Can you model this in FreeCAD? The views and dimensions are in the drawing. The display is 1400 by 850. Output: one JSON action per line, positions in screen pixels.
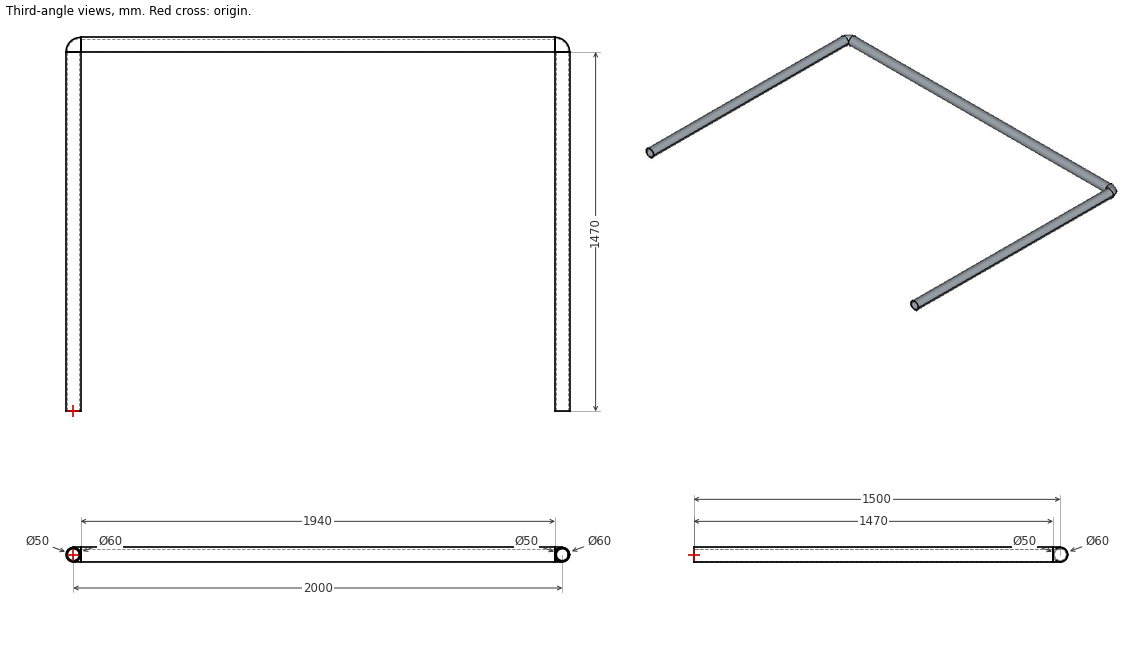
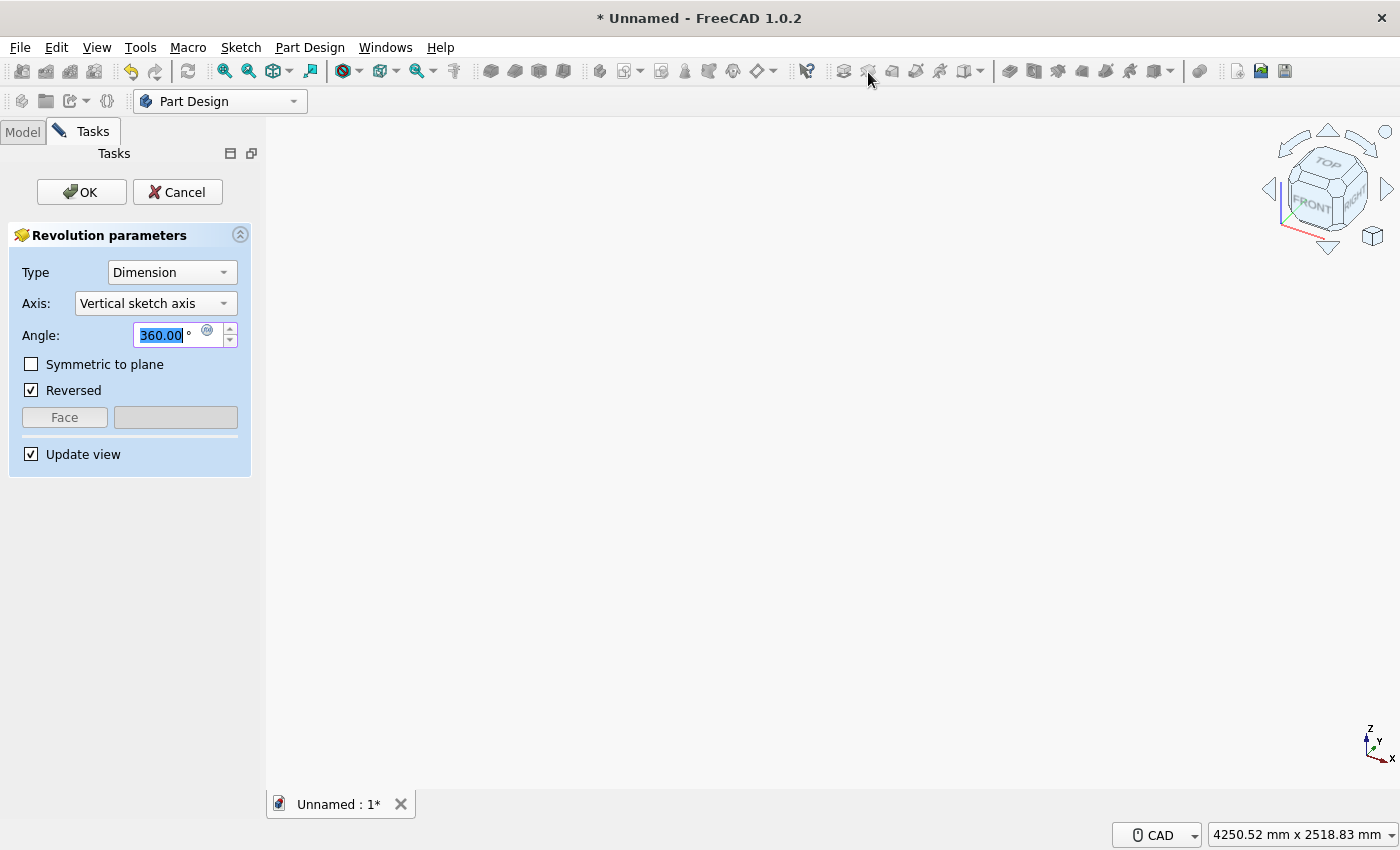
{"action": "left_click", "coordinate": [156, 304]}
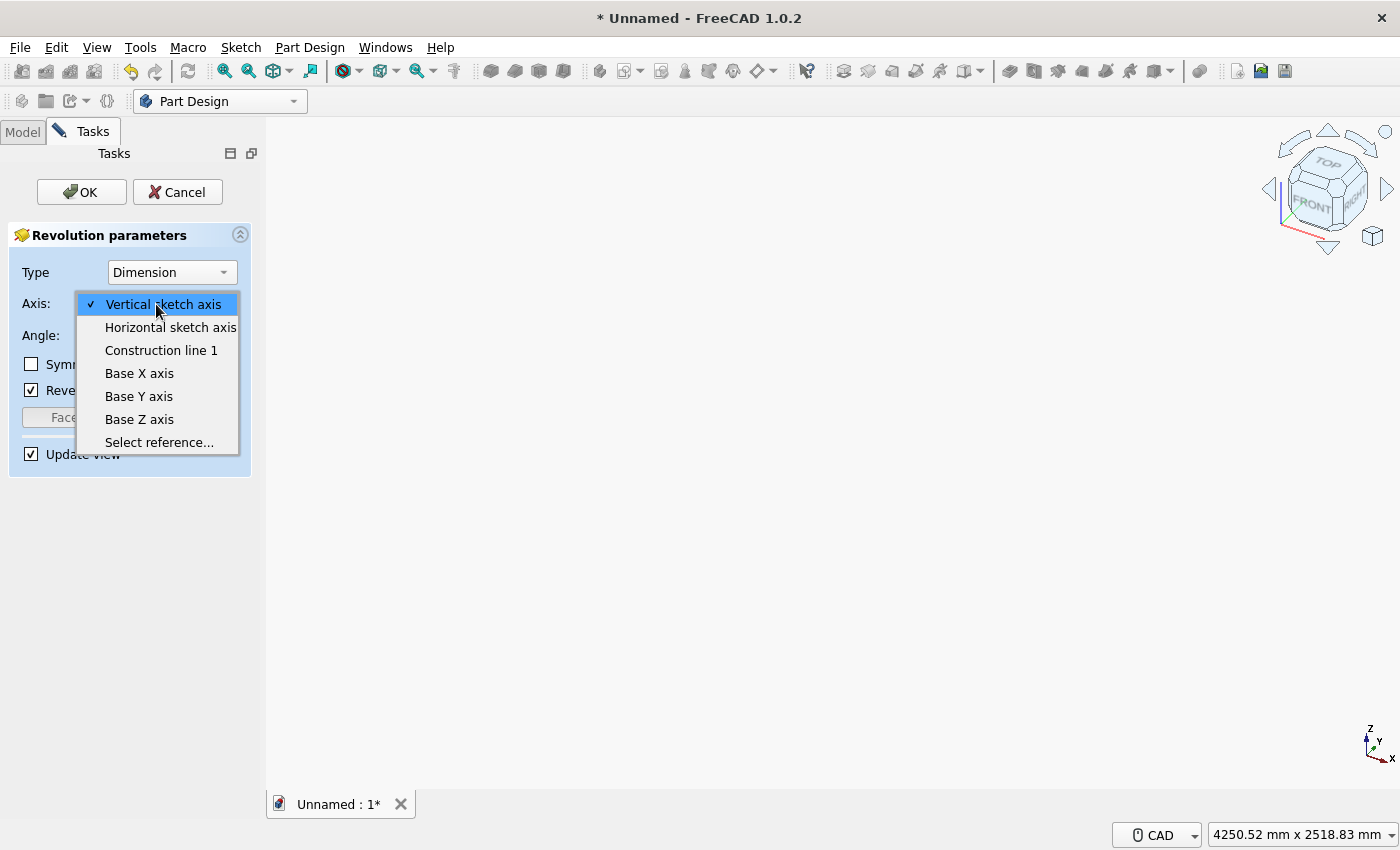
{"action": "left_click", "coordinate": [156, 350]}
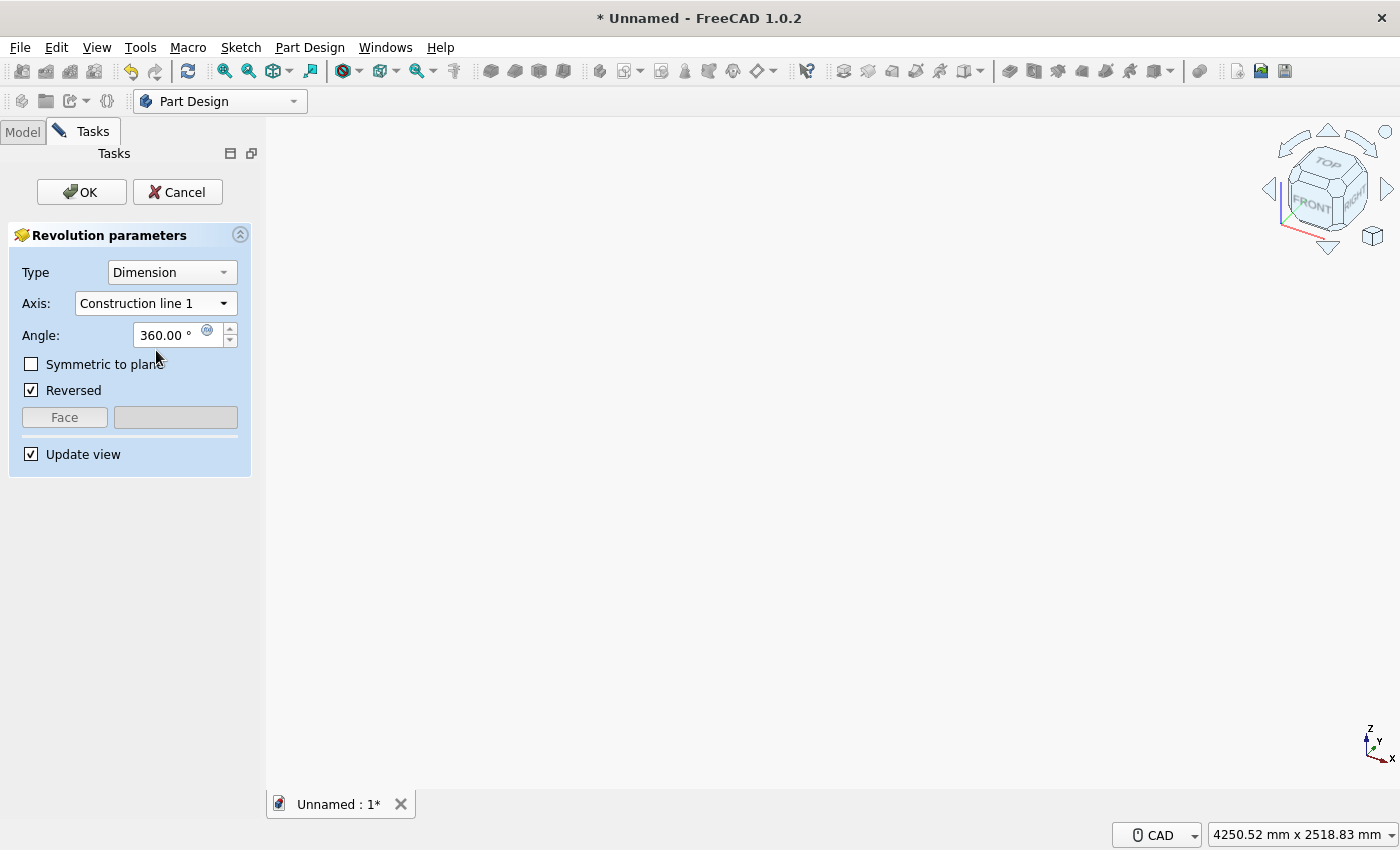
{"action": "triple_click", "coordinate": [178, 335]}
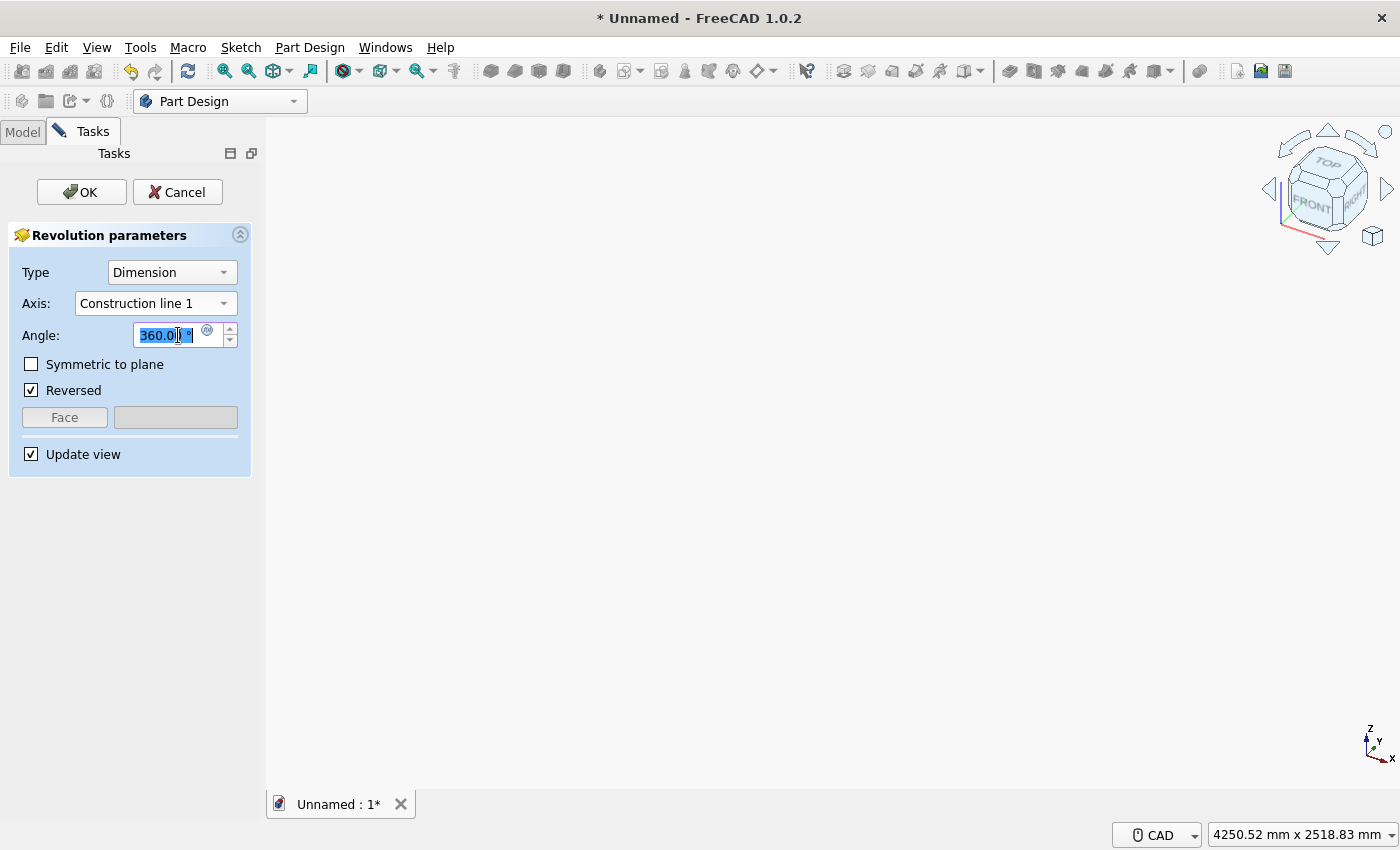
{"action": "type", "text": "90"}
{"action": "key", "text": "Tab"}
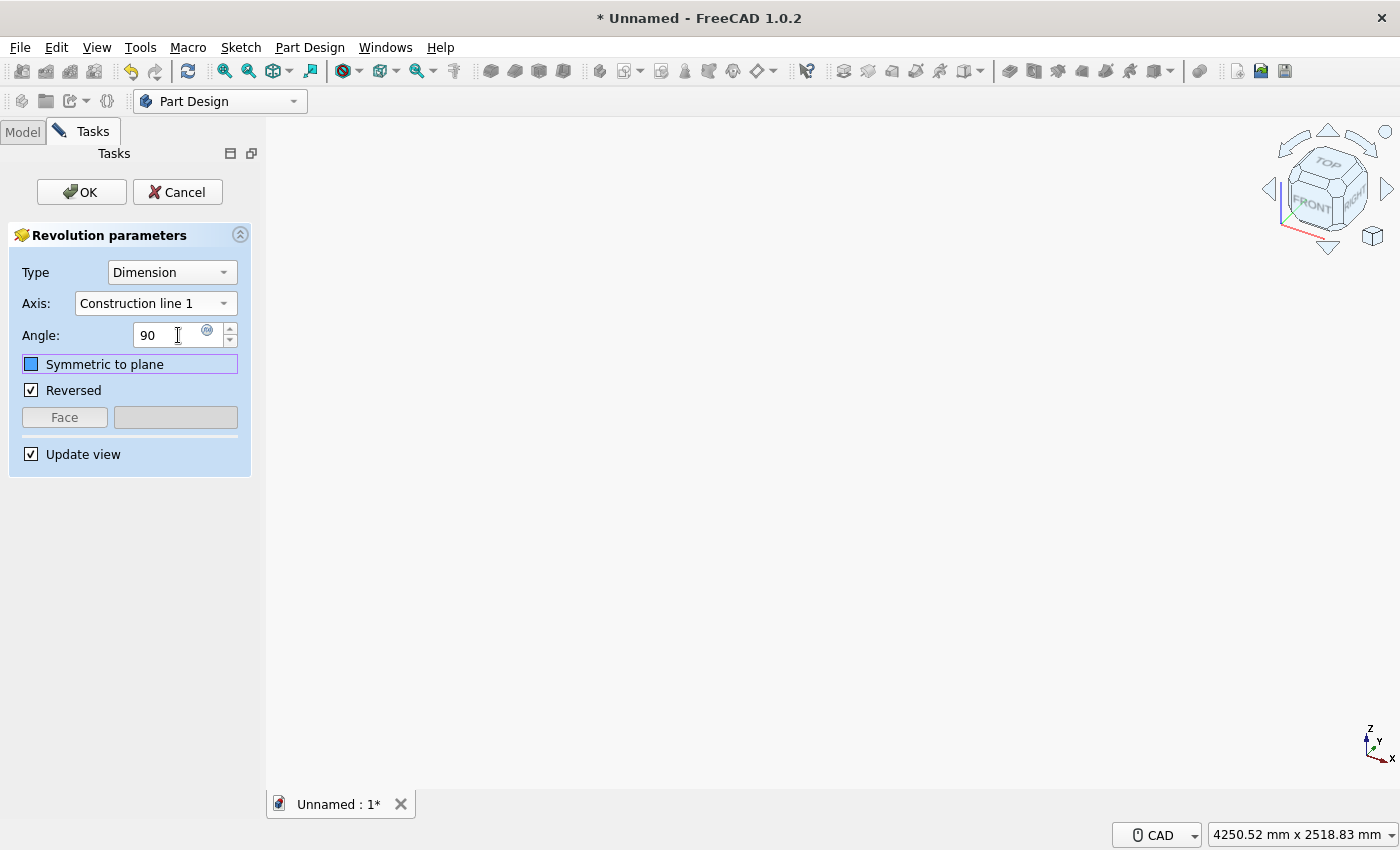
{"action": "left_click", "coordinate": [30, 390]}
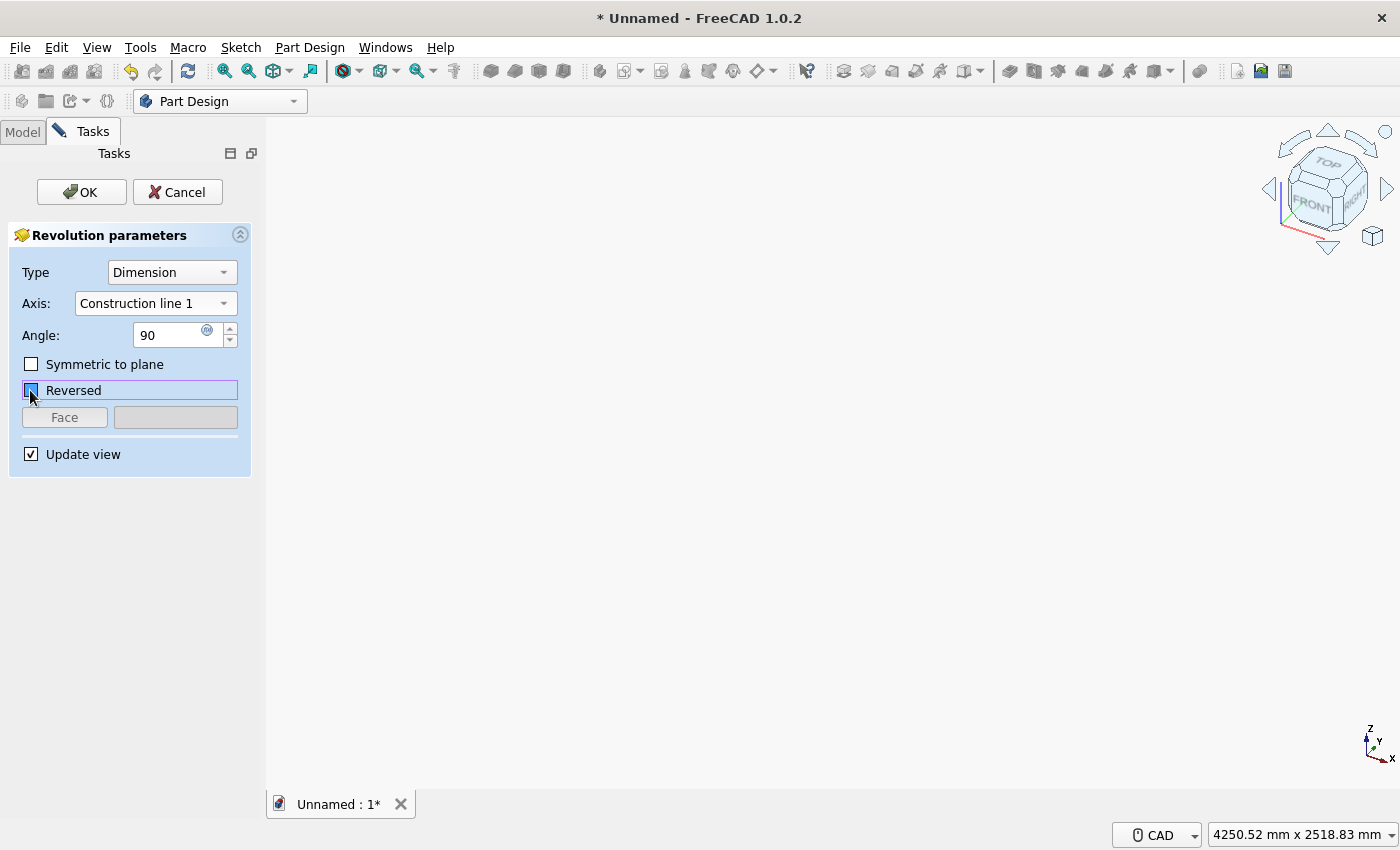
{"action": "left_click", "coordinate": [82, 192]}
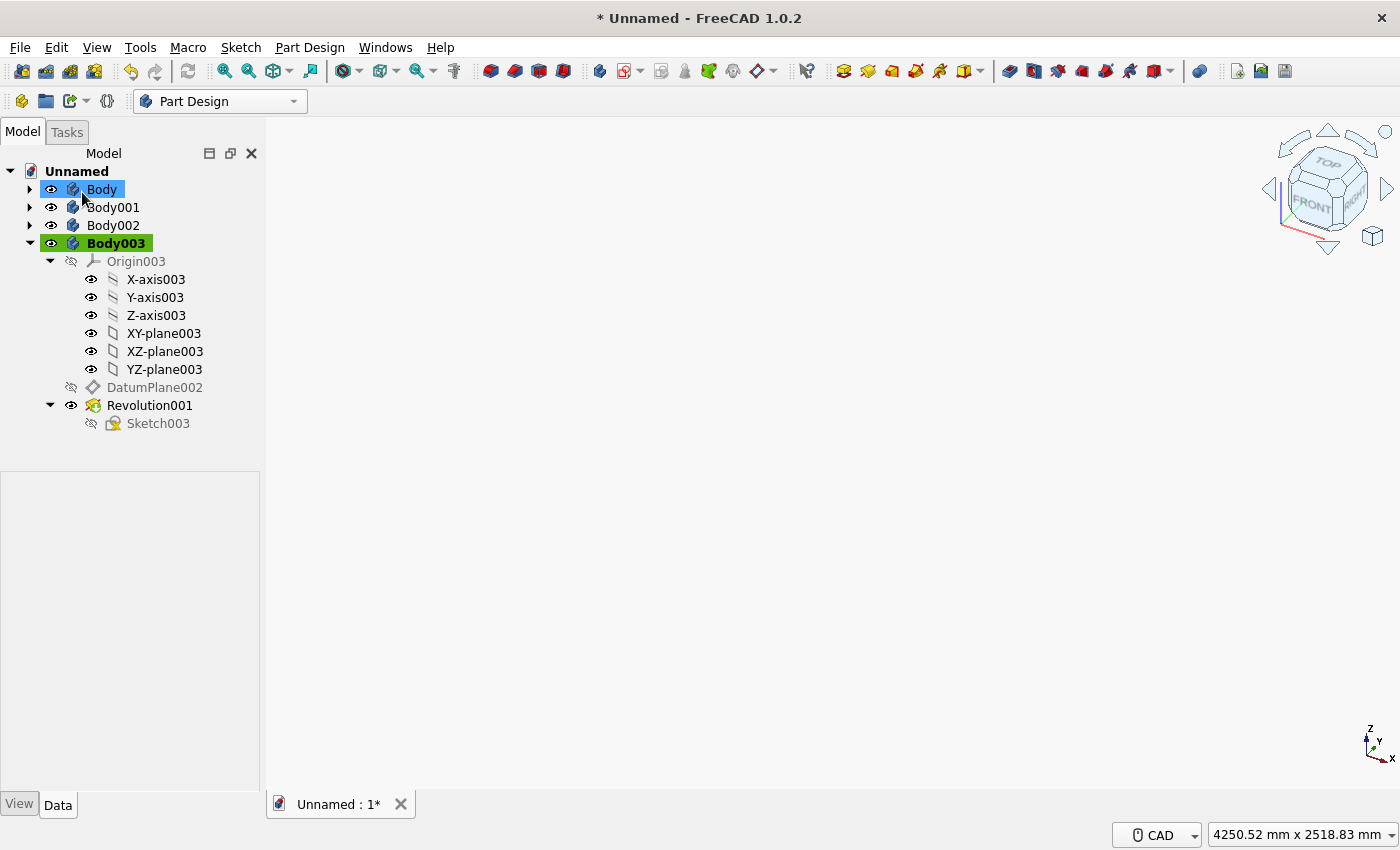
{"action": "left_click", "coordinate": [226, 72]}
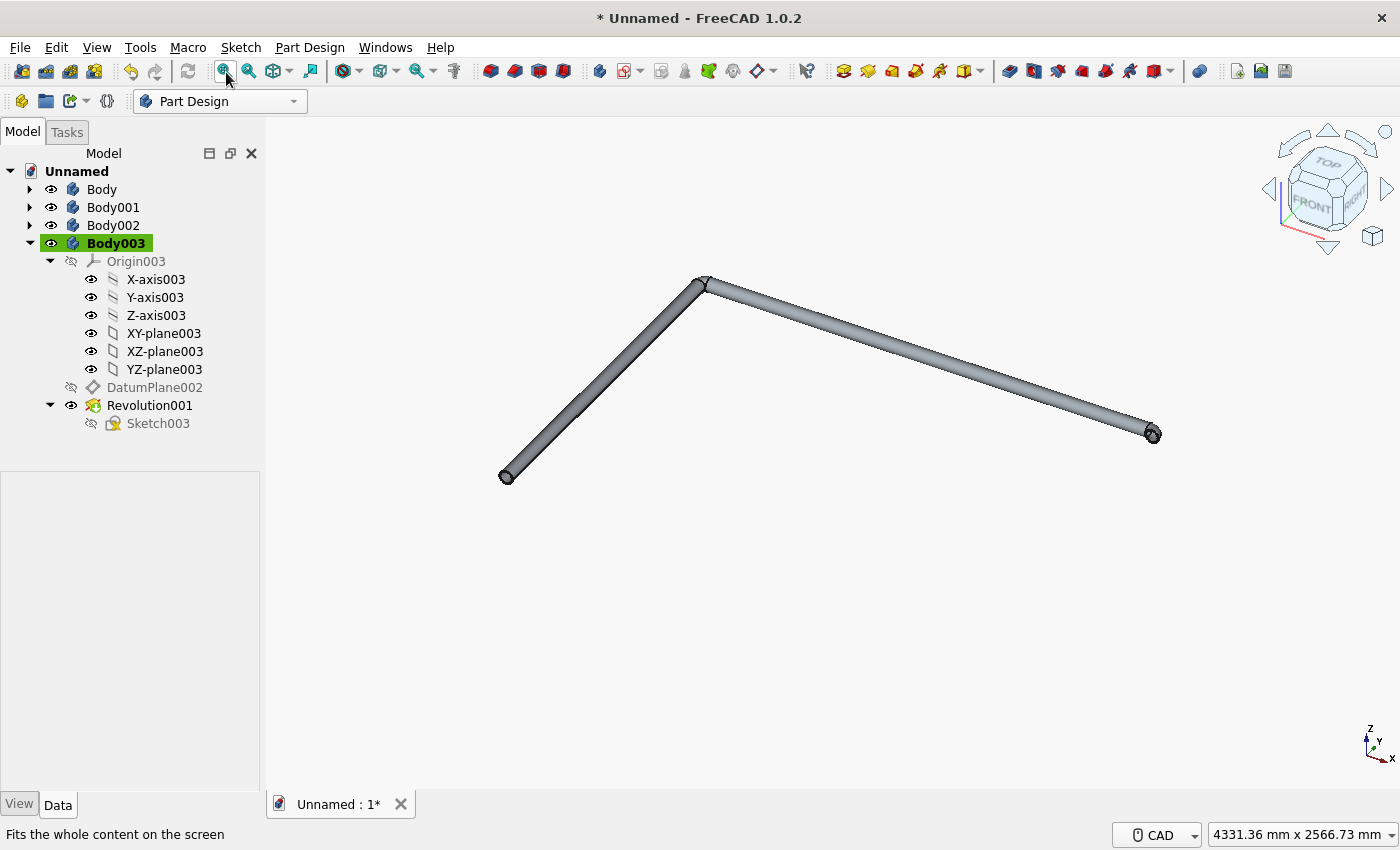
{"action": "left_click", "coordinate": [600, 72]}